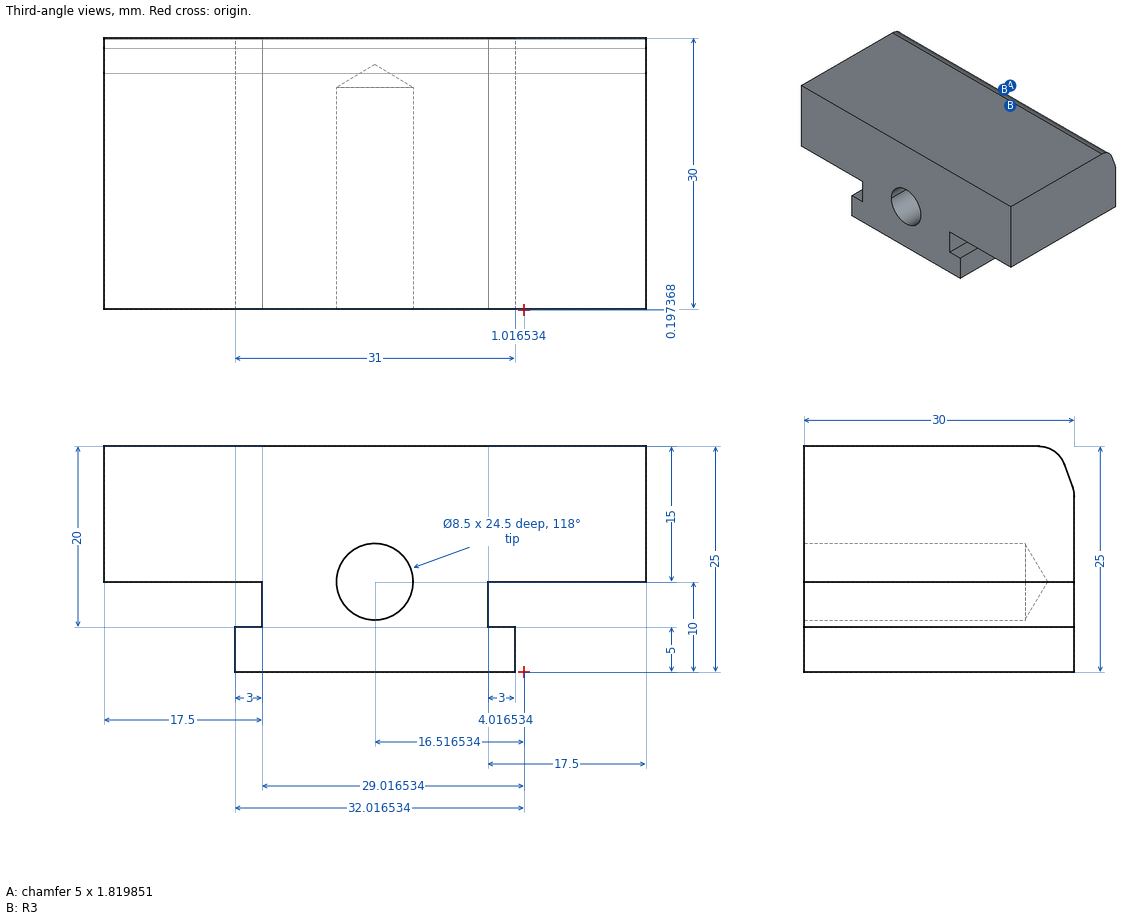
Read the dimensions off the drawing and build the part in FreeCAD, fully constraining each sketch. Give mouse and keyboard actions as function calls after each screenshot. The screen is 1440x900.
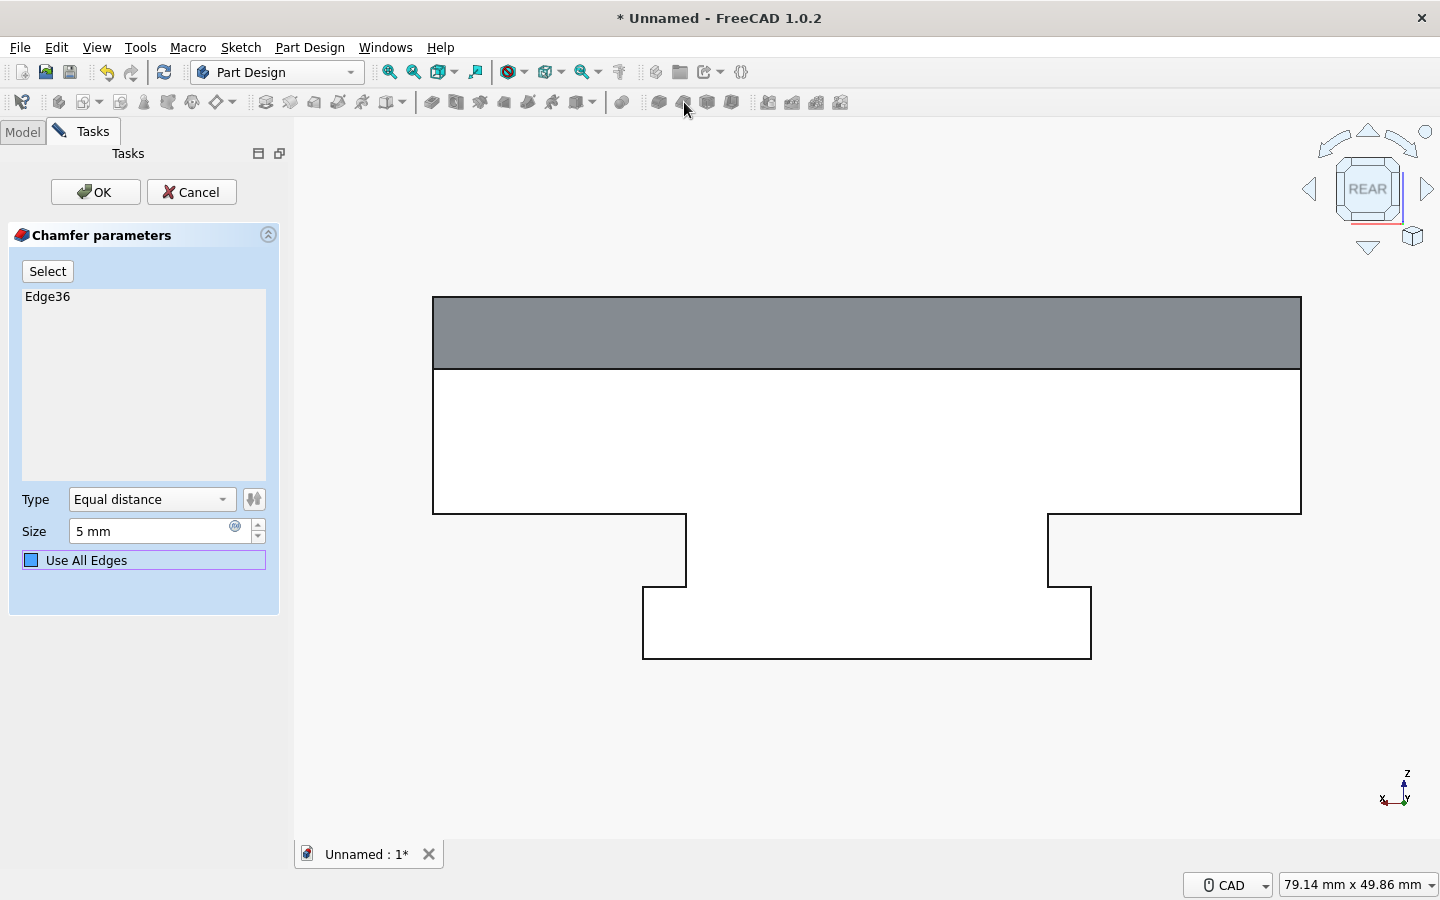
click(153, 500)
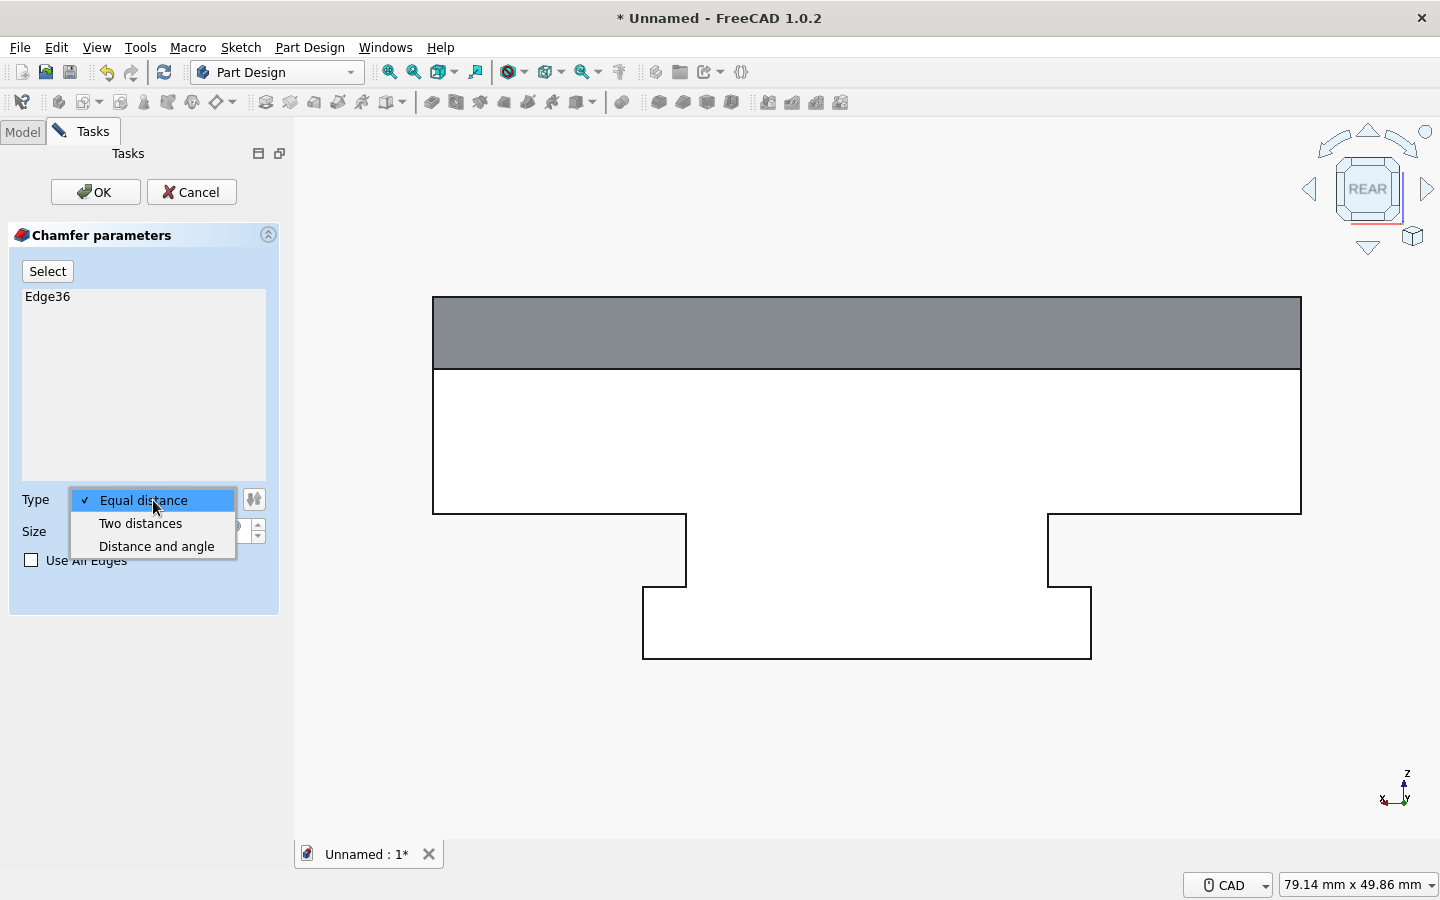
click(152, 524)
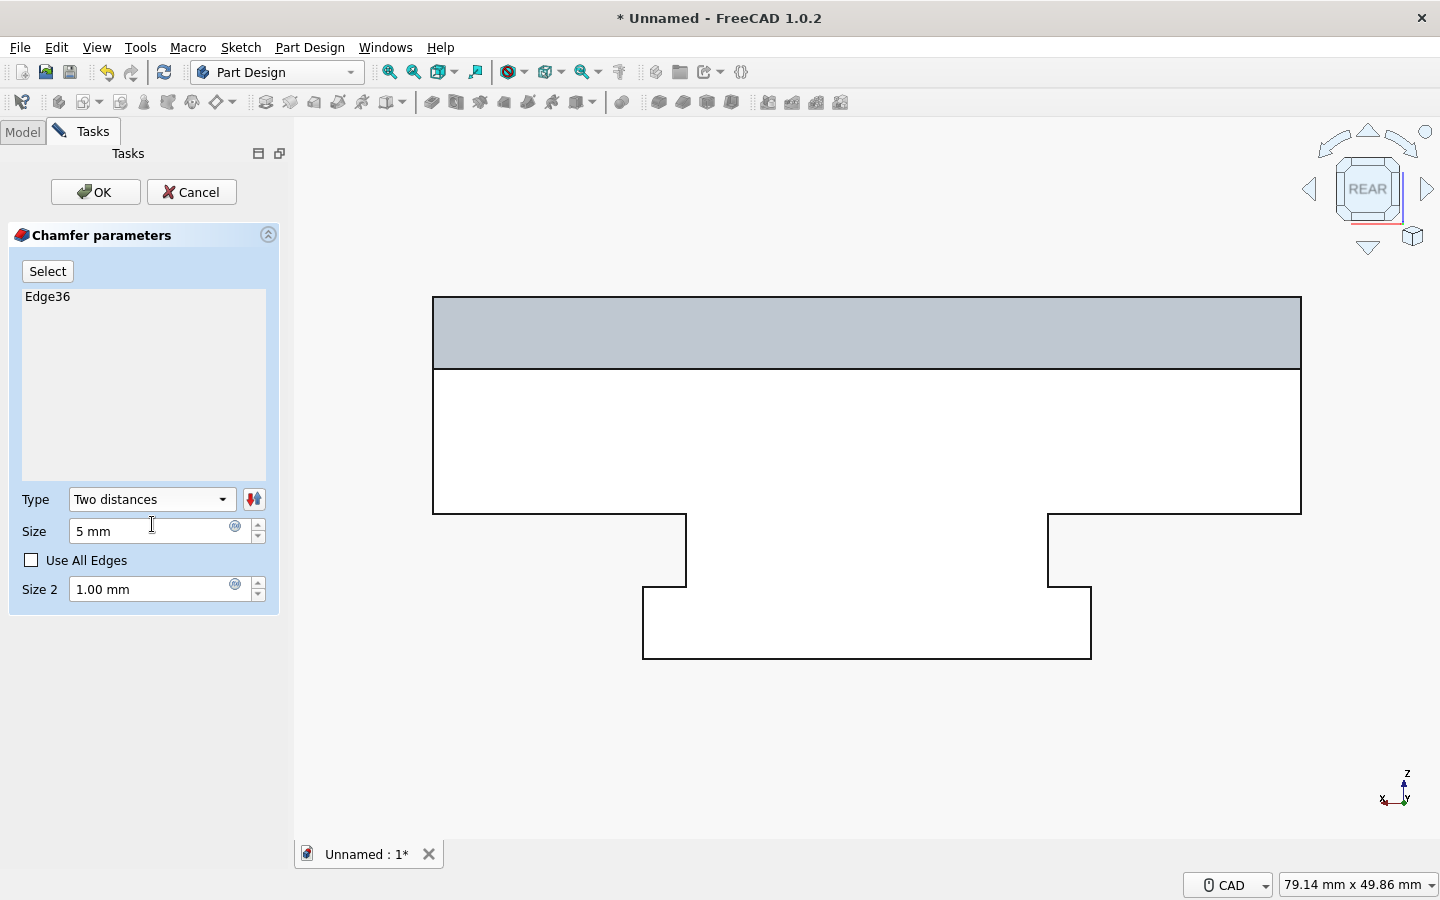
triple_click(160, 589)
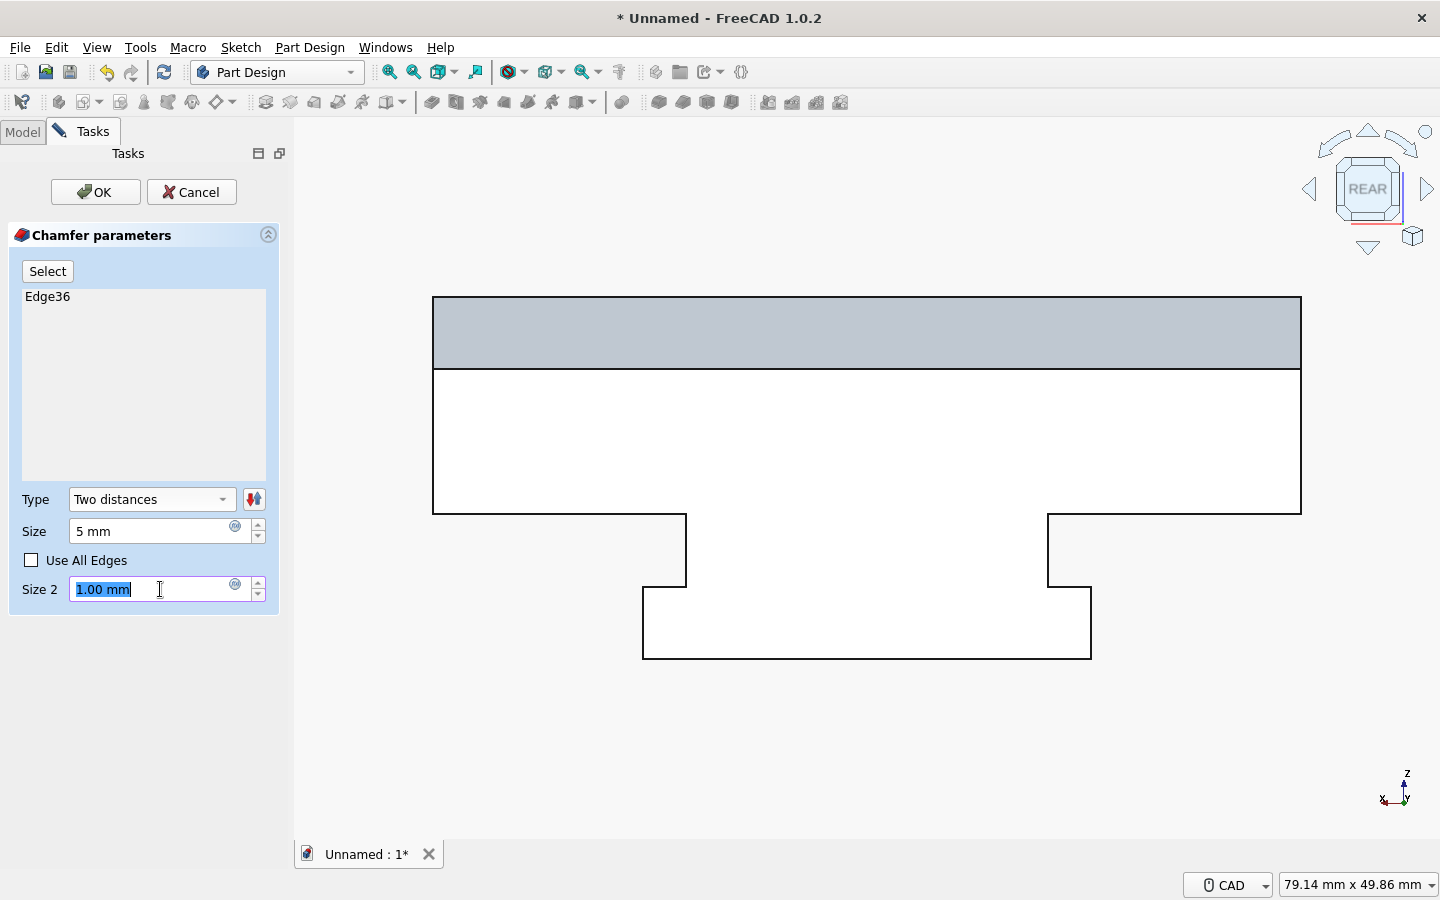
text(1.819851)
key(Tab)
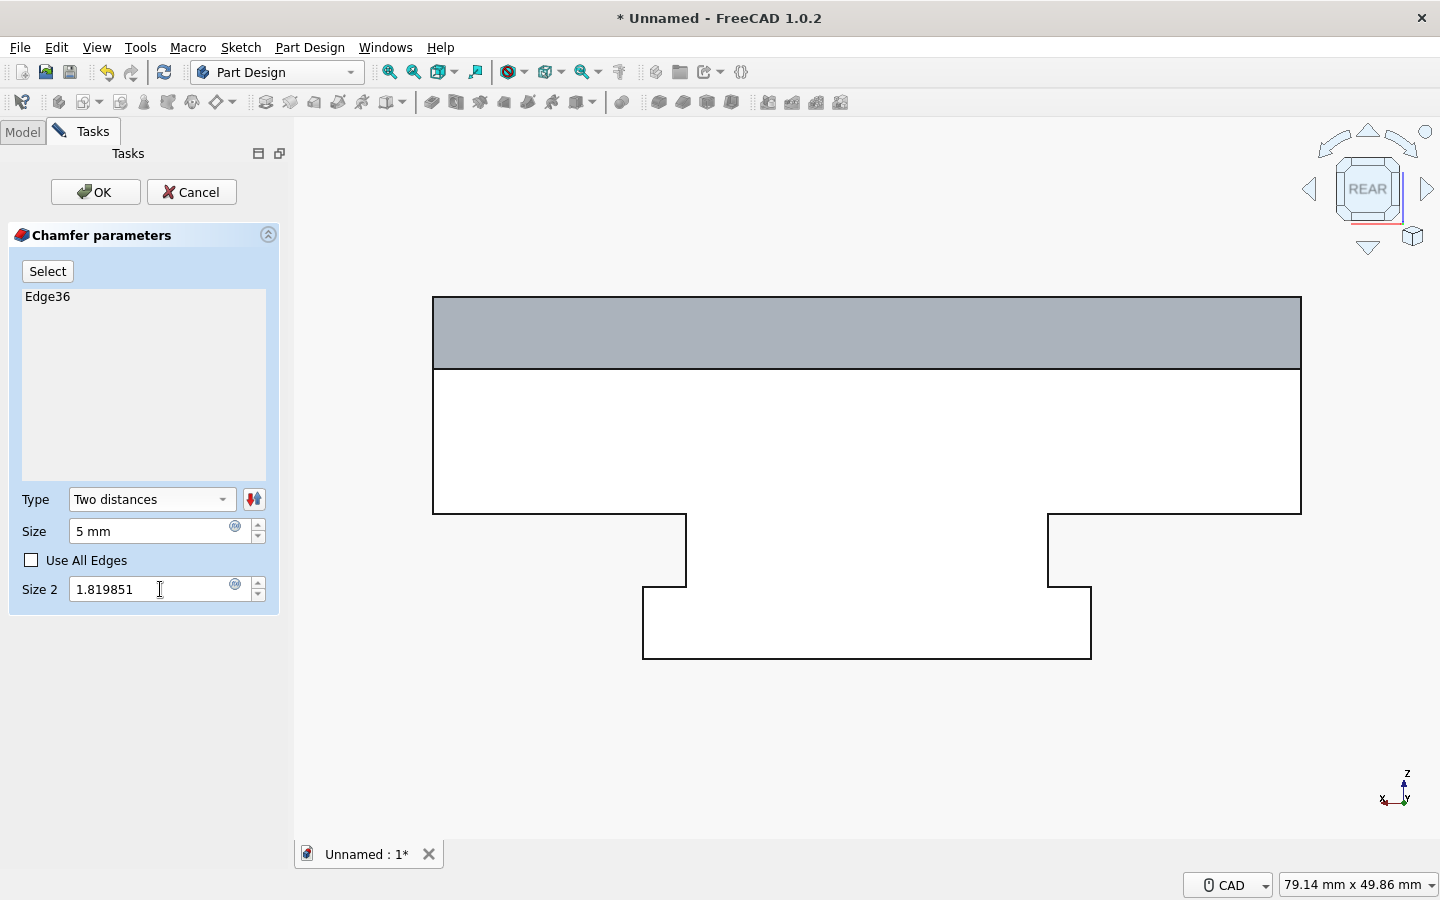
click(96, 192)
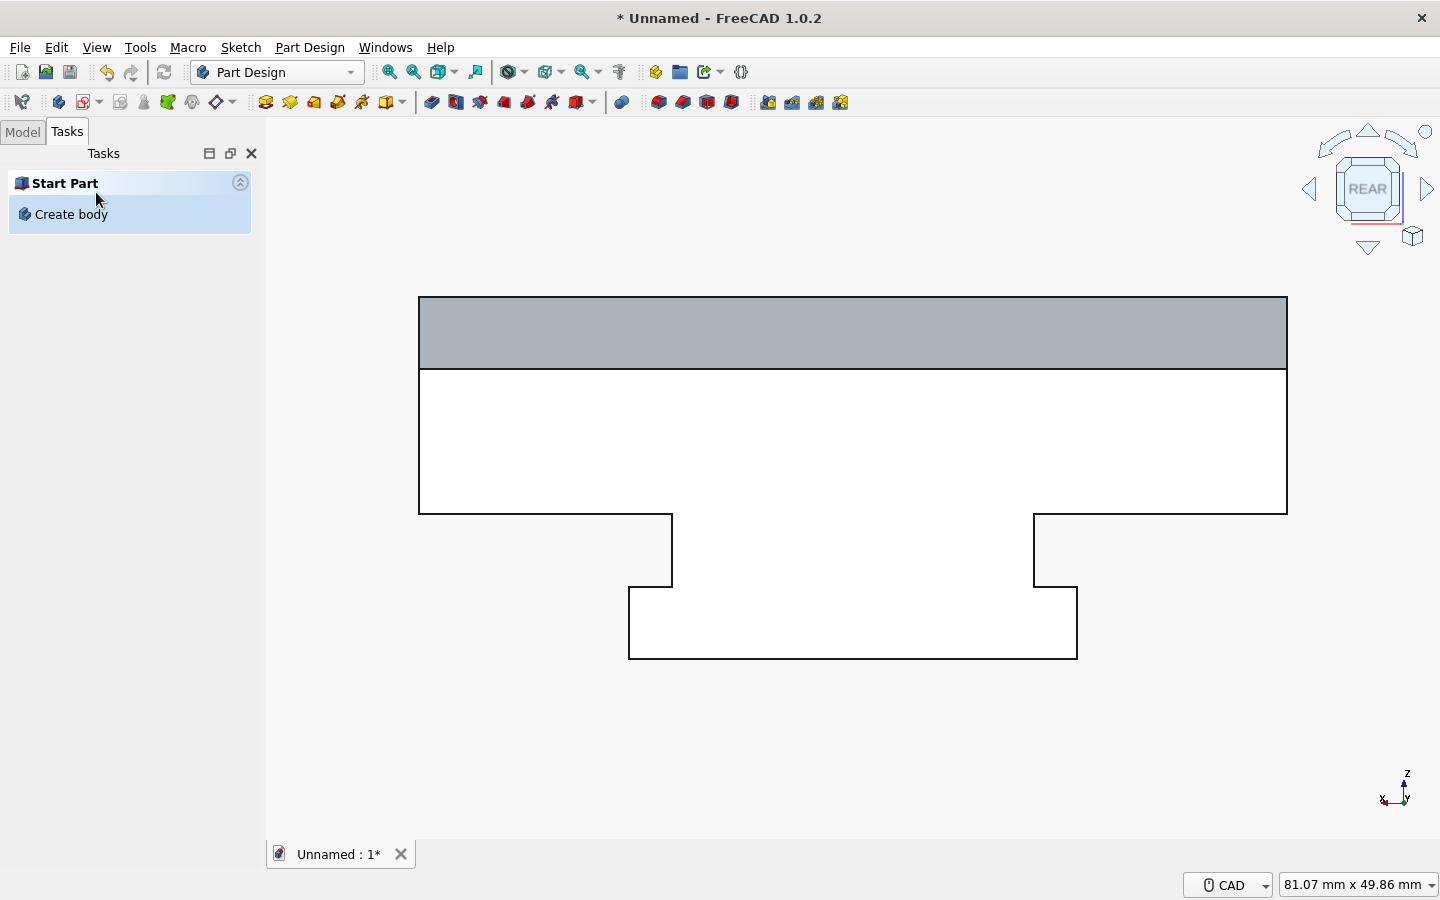
click(853, 368)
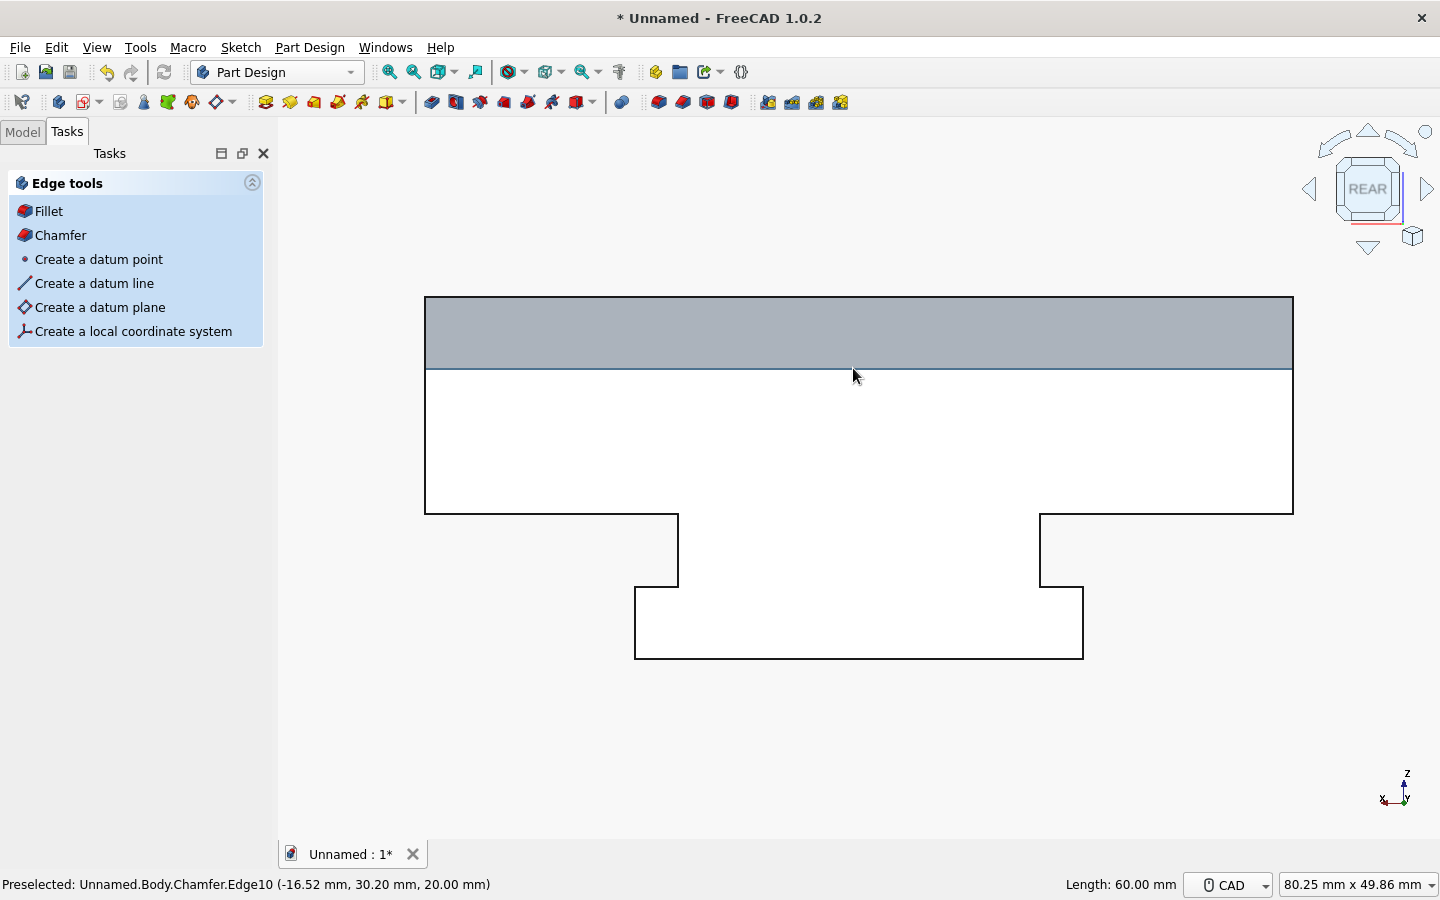
key(0)